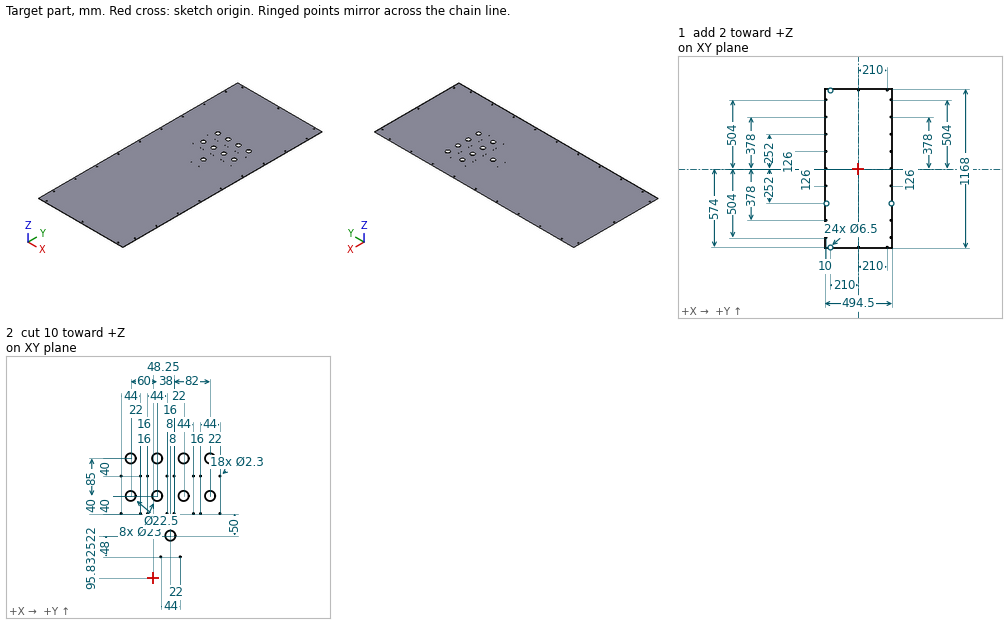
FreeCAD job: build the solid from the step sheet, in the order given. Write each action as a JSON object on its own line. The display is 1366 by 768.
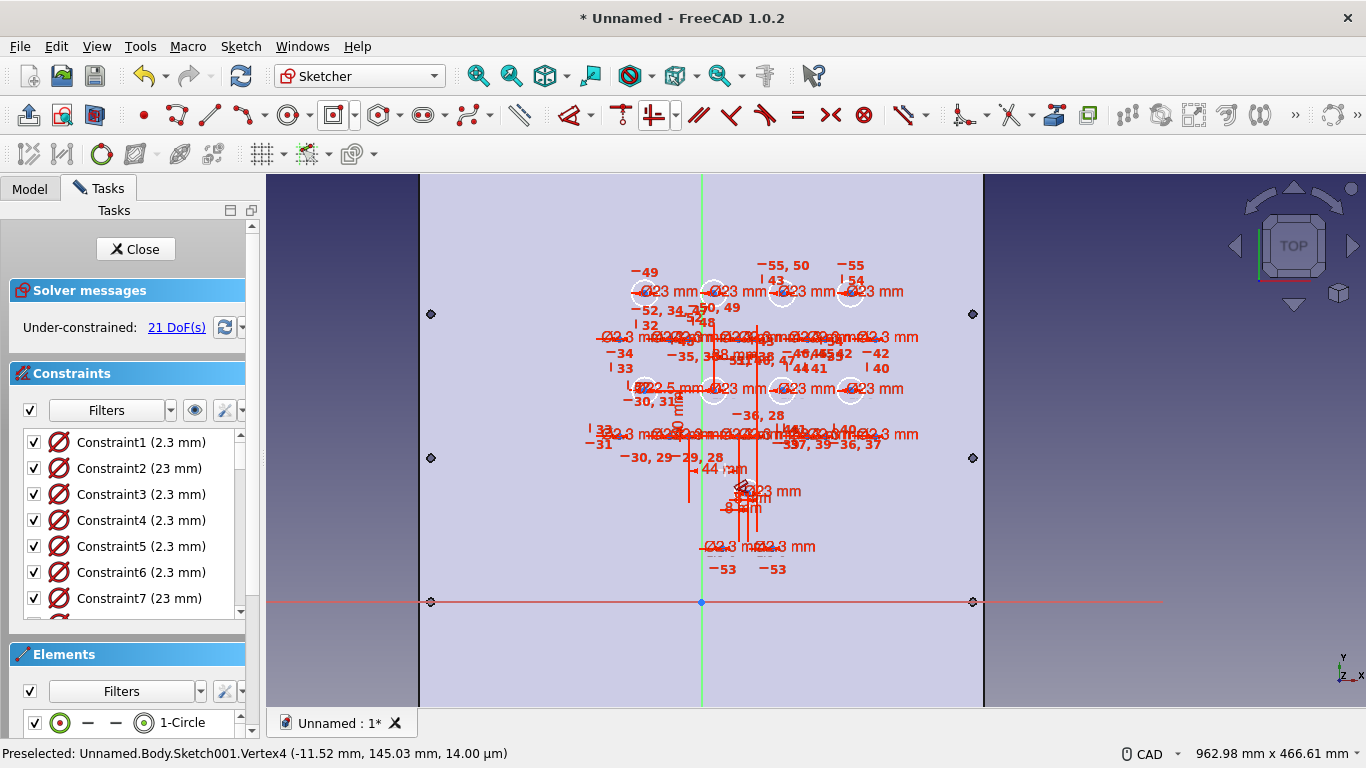
{"action": "scroll", "coordinate": [689, 436], "scroll_direction": "up", "scroll_amount": 4}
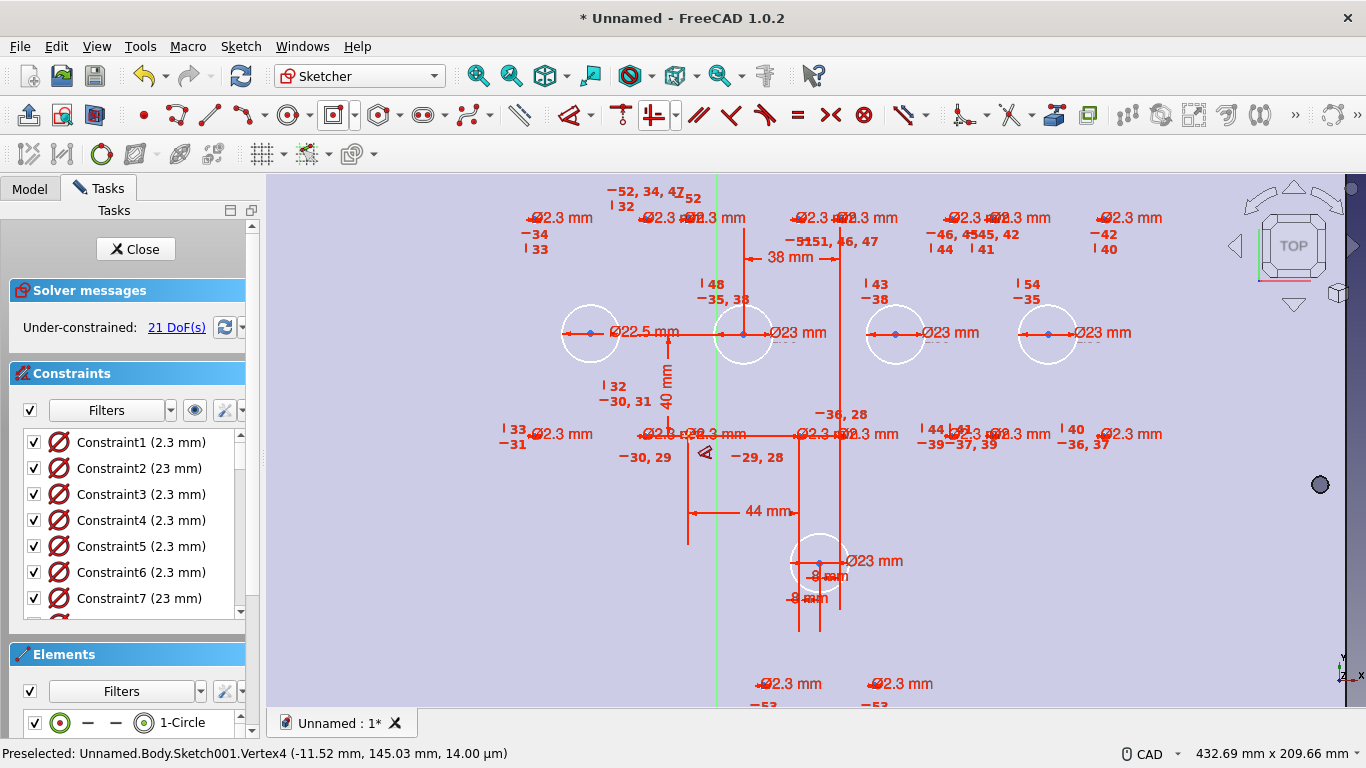
{"action": "left_click", "coordinate": [688, 436]}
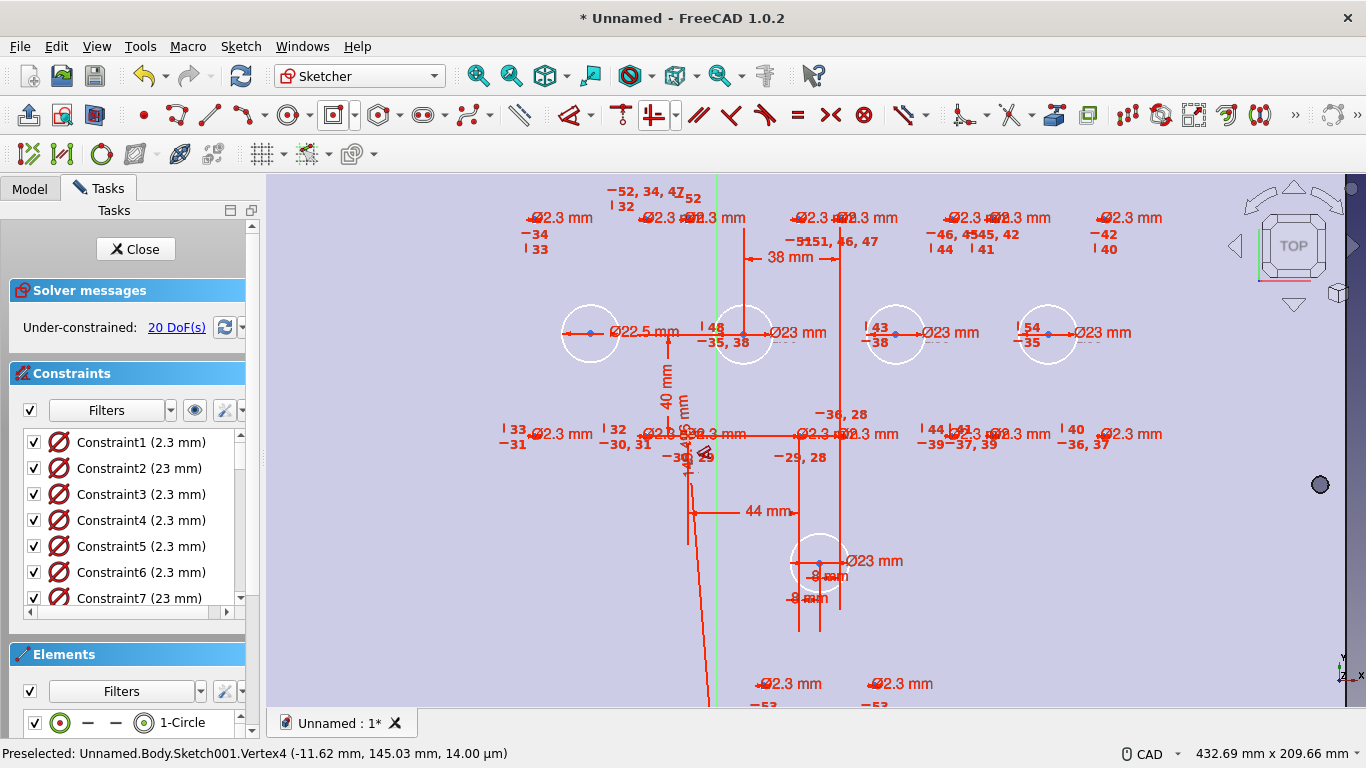
{"action": "left_click", "coordinate": [646, 436]}
{"action": "left_click", "coordinate": [667, 470]}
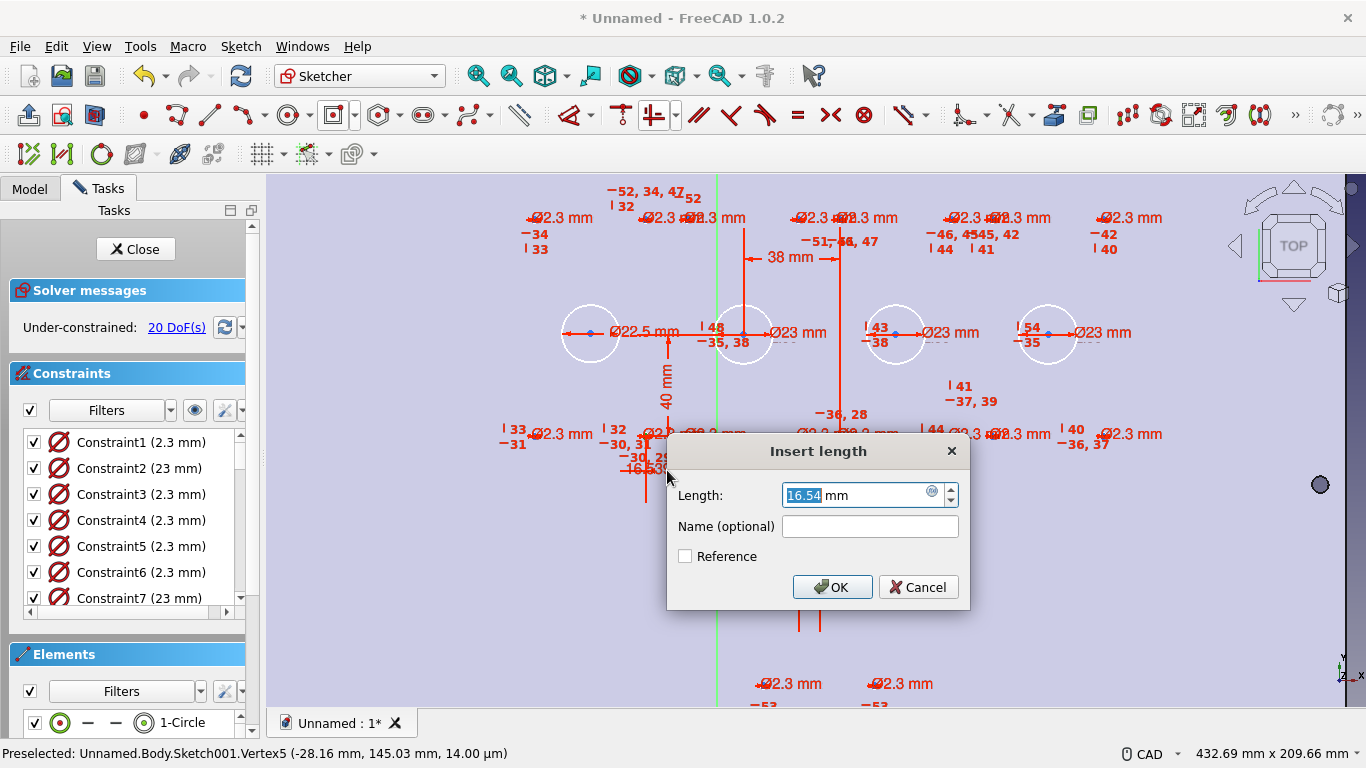
{"action": "type", "text": "16"}
{"action": "key", "text": "Return"}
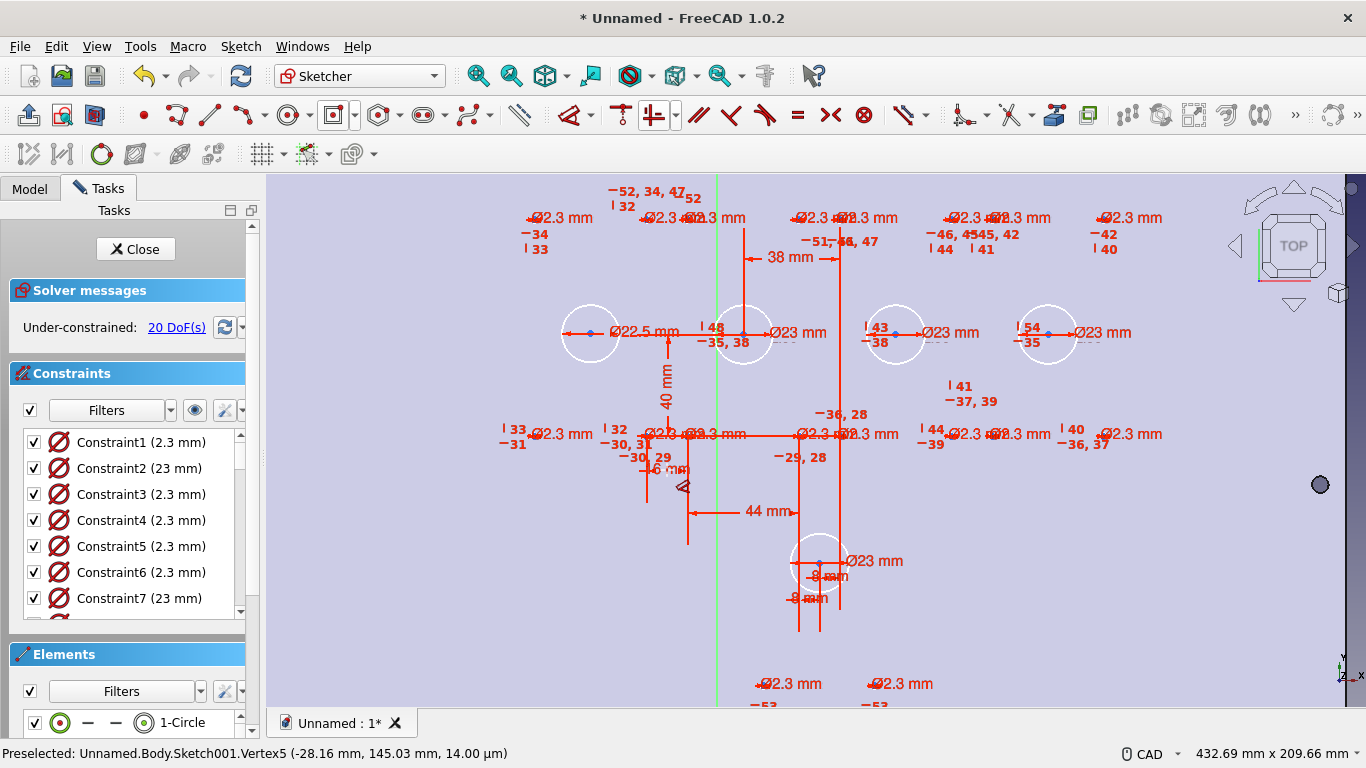
{"action": "left_click", "coordinate": [647, 436]}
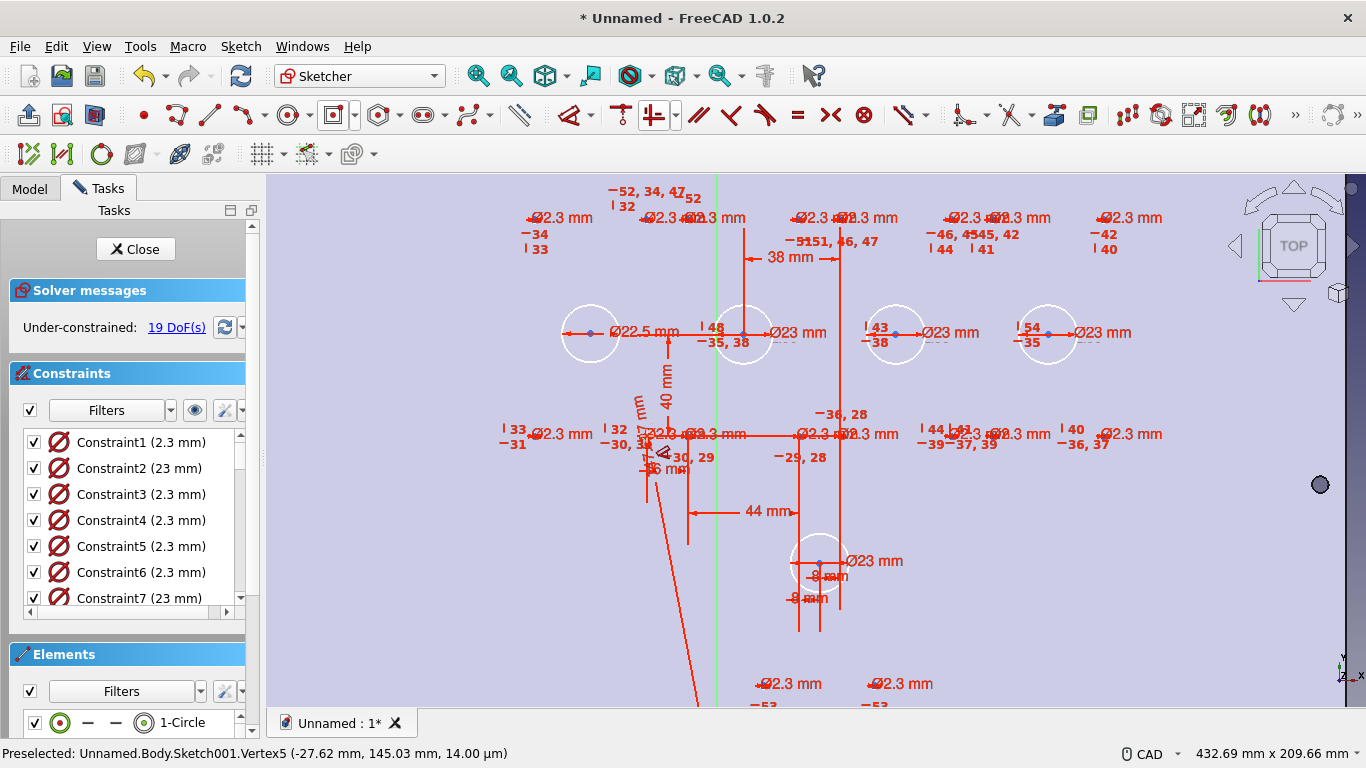
{"action": "left_click", "coordinate": [534, 436]}
{"action": "left_click", "coordinate": [591, 402]}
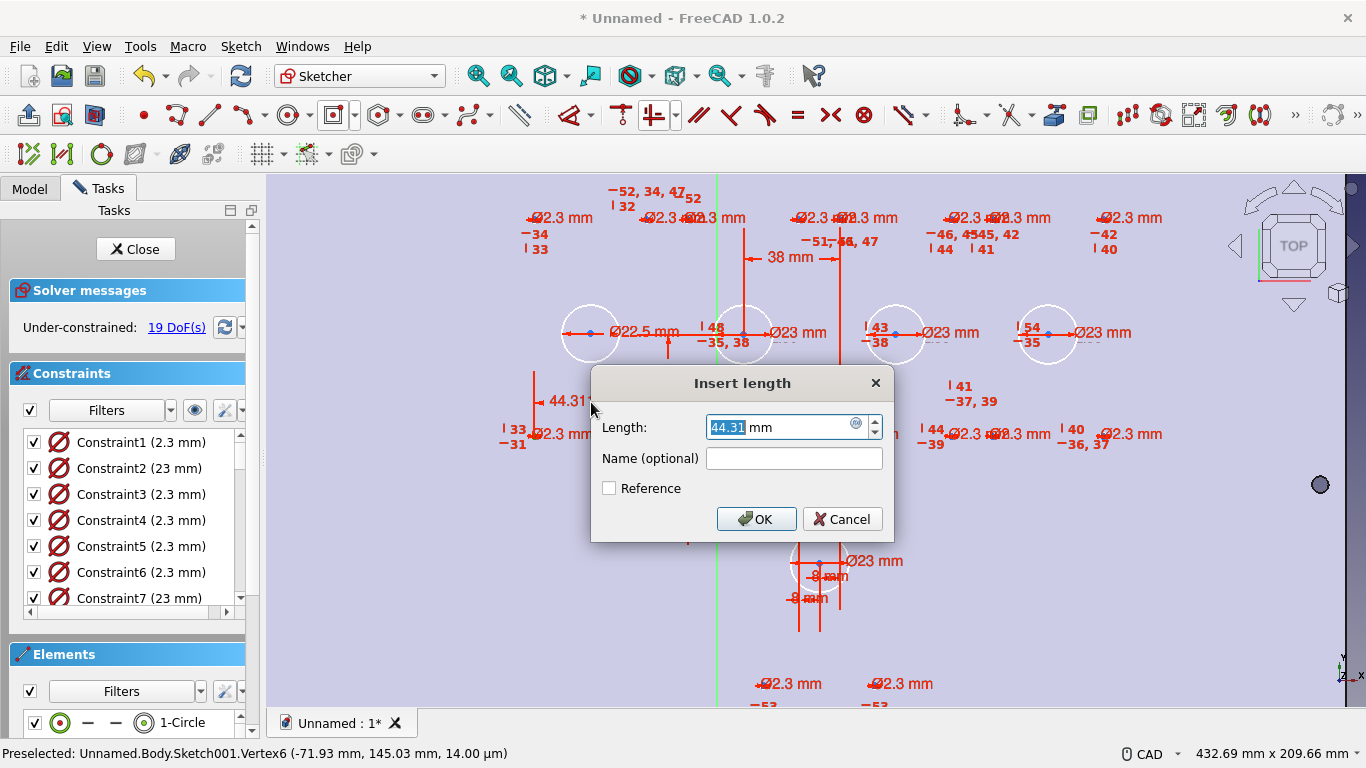
{"action": "type", "text": "44"}
{"action": "key", "text": "Return"}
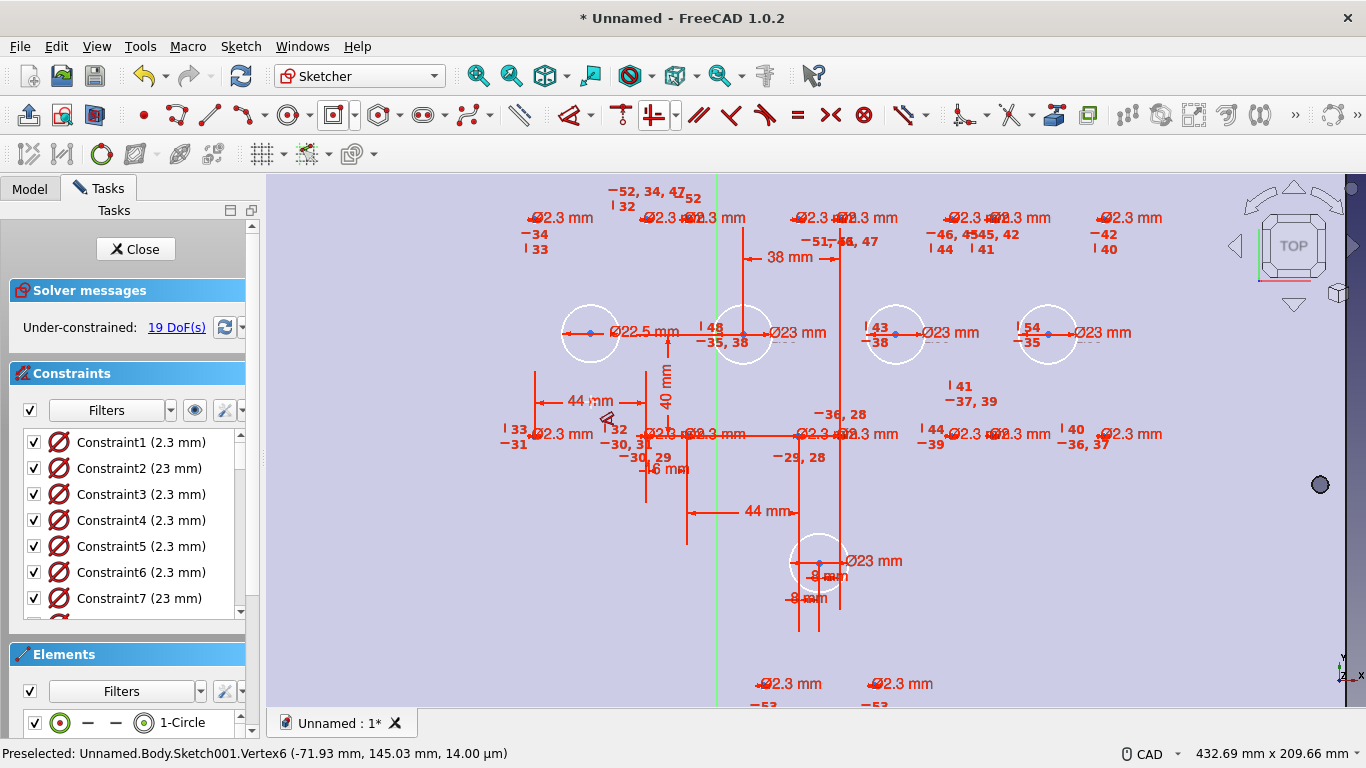
{"action": "left_click", "coordinate": [743, 335]}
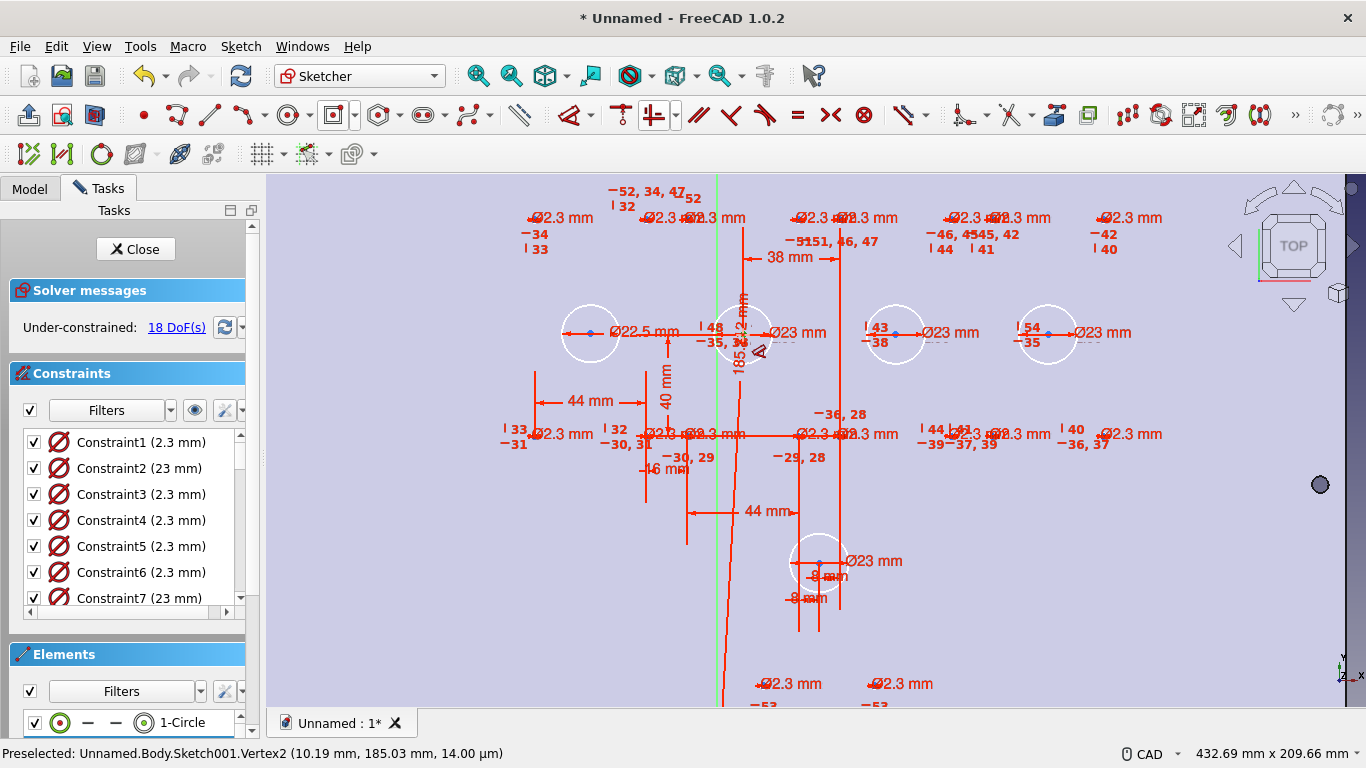
{"action": "scroll", "coordinate": [689, 436], "scroll_direction": "down", "scroll_amount": 4}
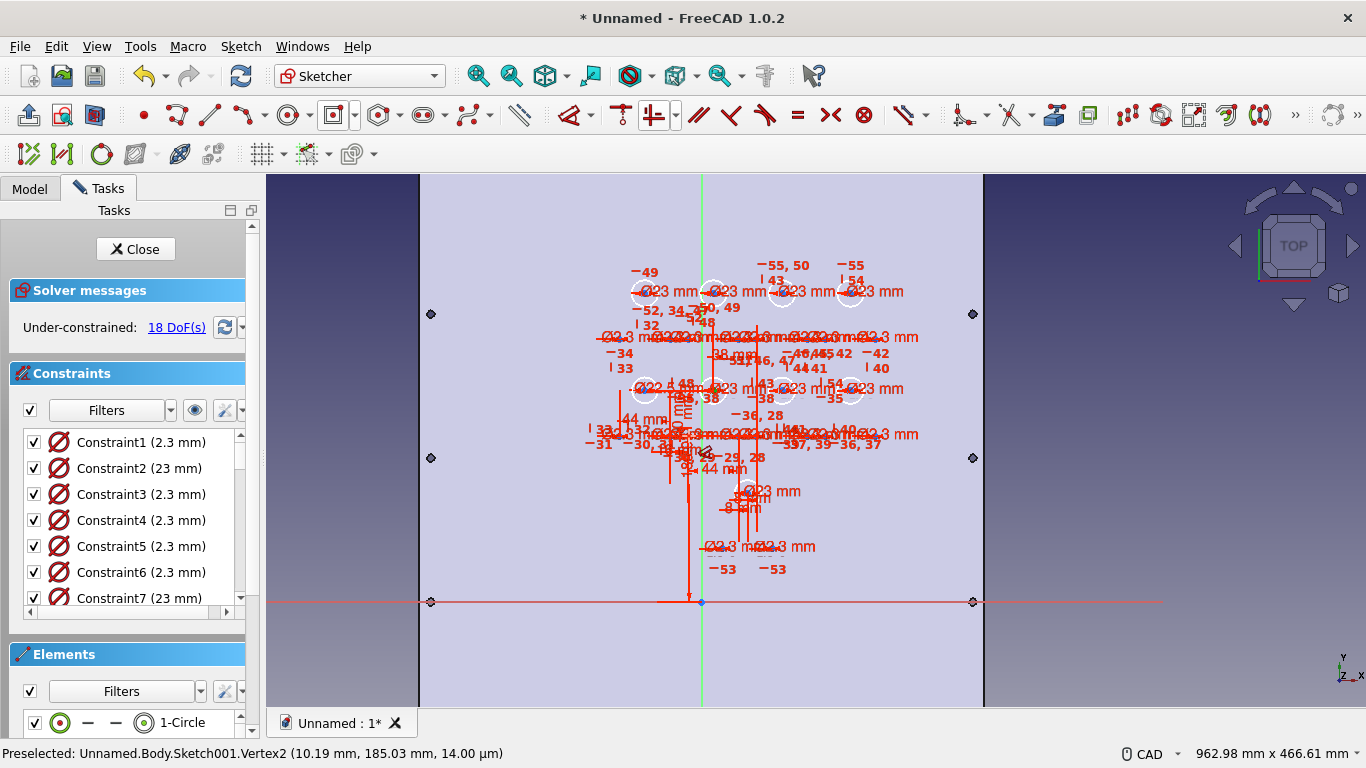
{"action": "left_click", "coordinate": [645, 293]}
{"action": "left_click", "coordinate": [679, 259]}